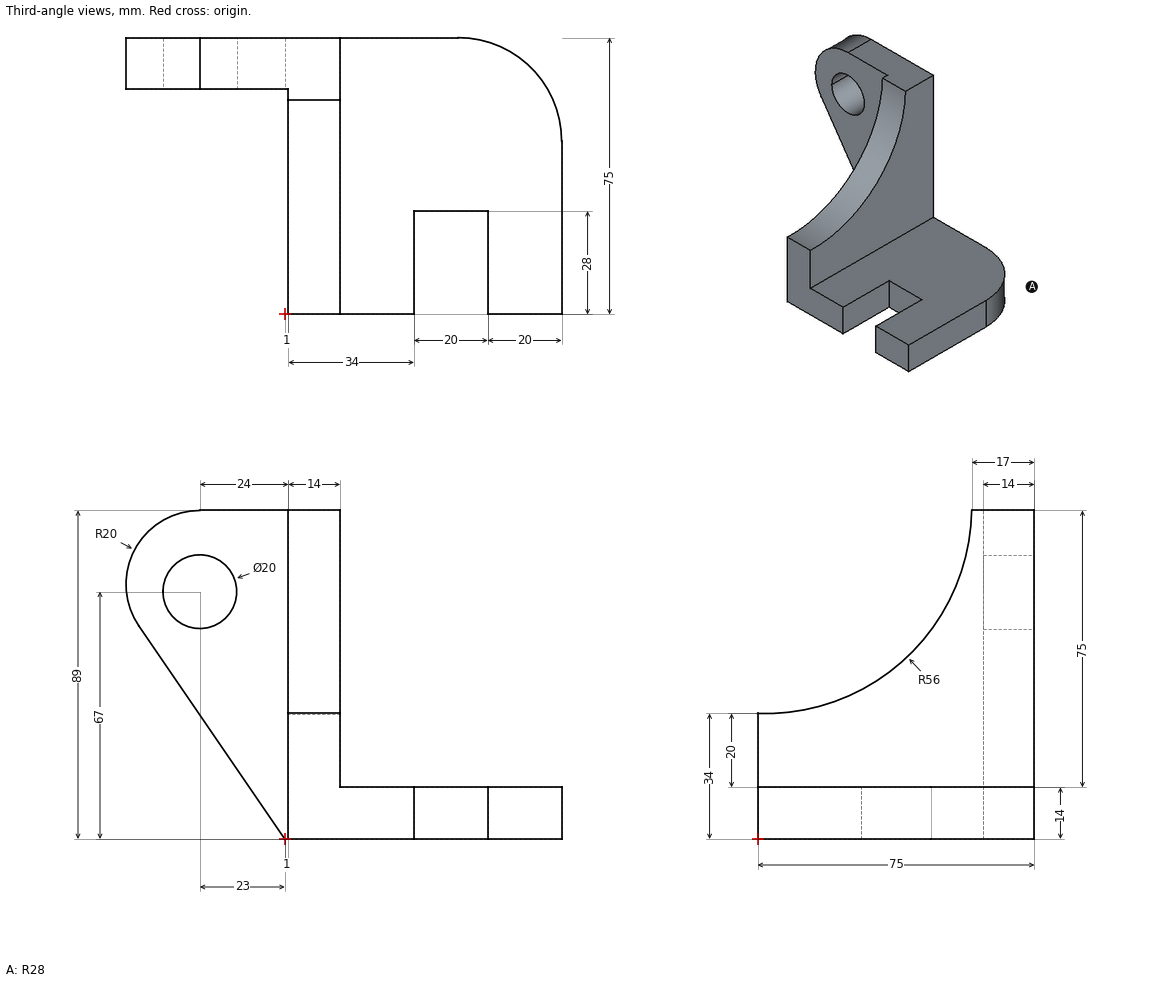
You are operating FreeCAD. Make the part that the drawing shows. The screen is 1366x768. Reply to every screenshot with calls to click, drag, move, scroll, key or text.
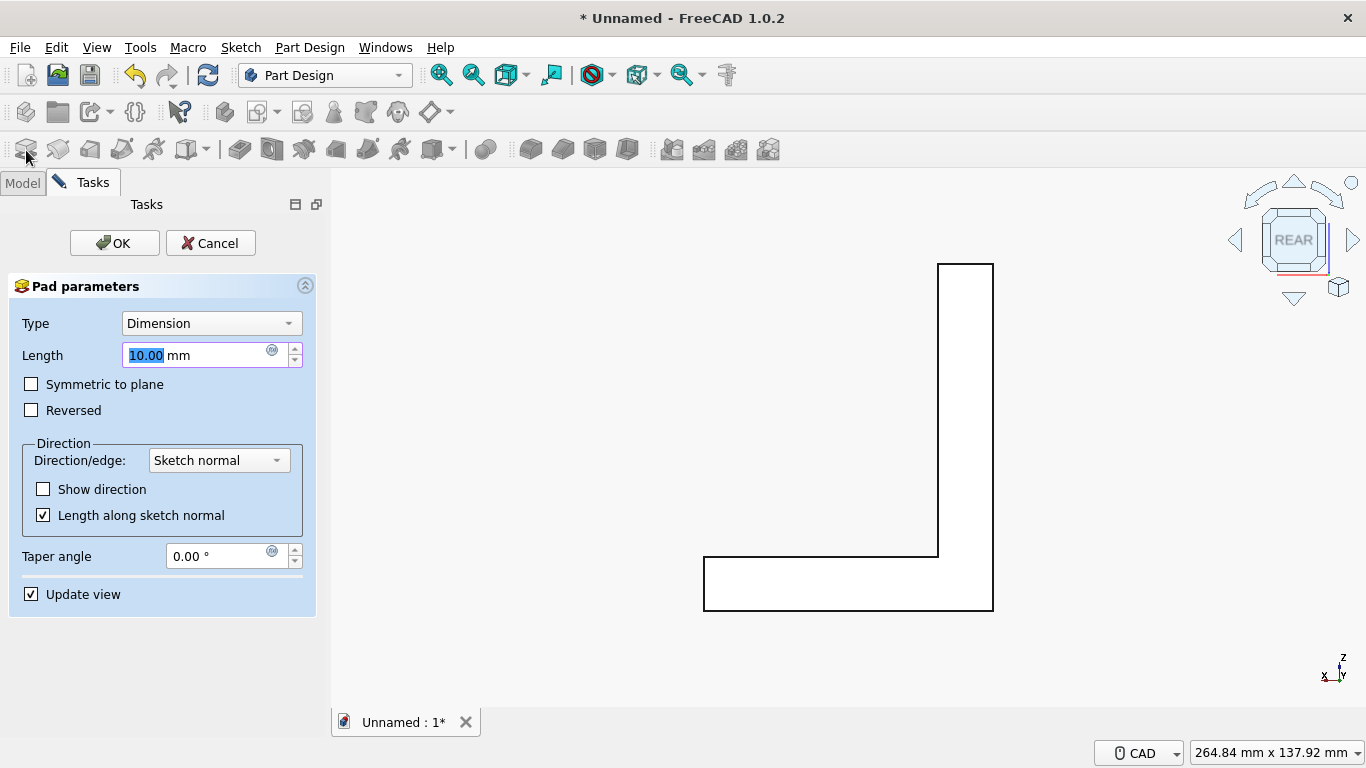
text(14)
key(Tab)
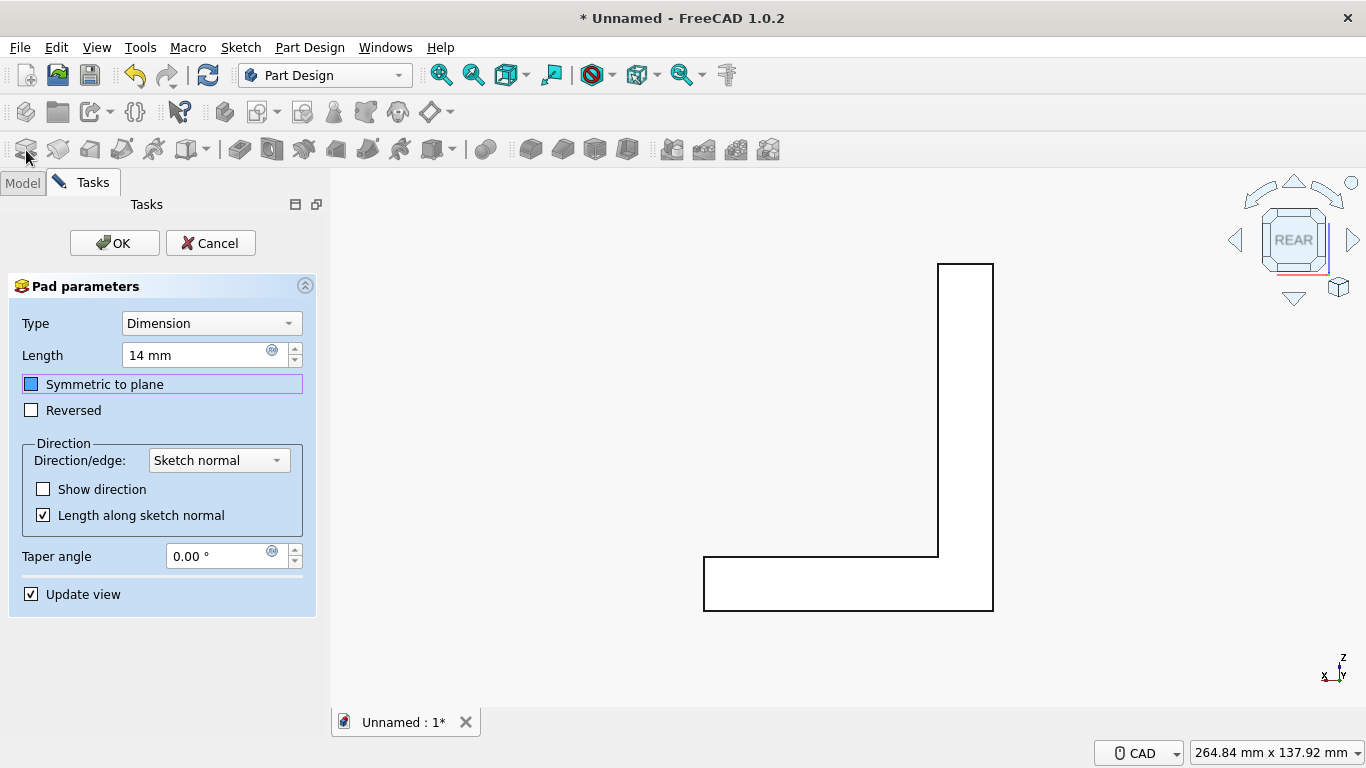
click(30, 410)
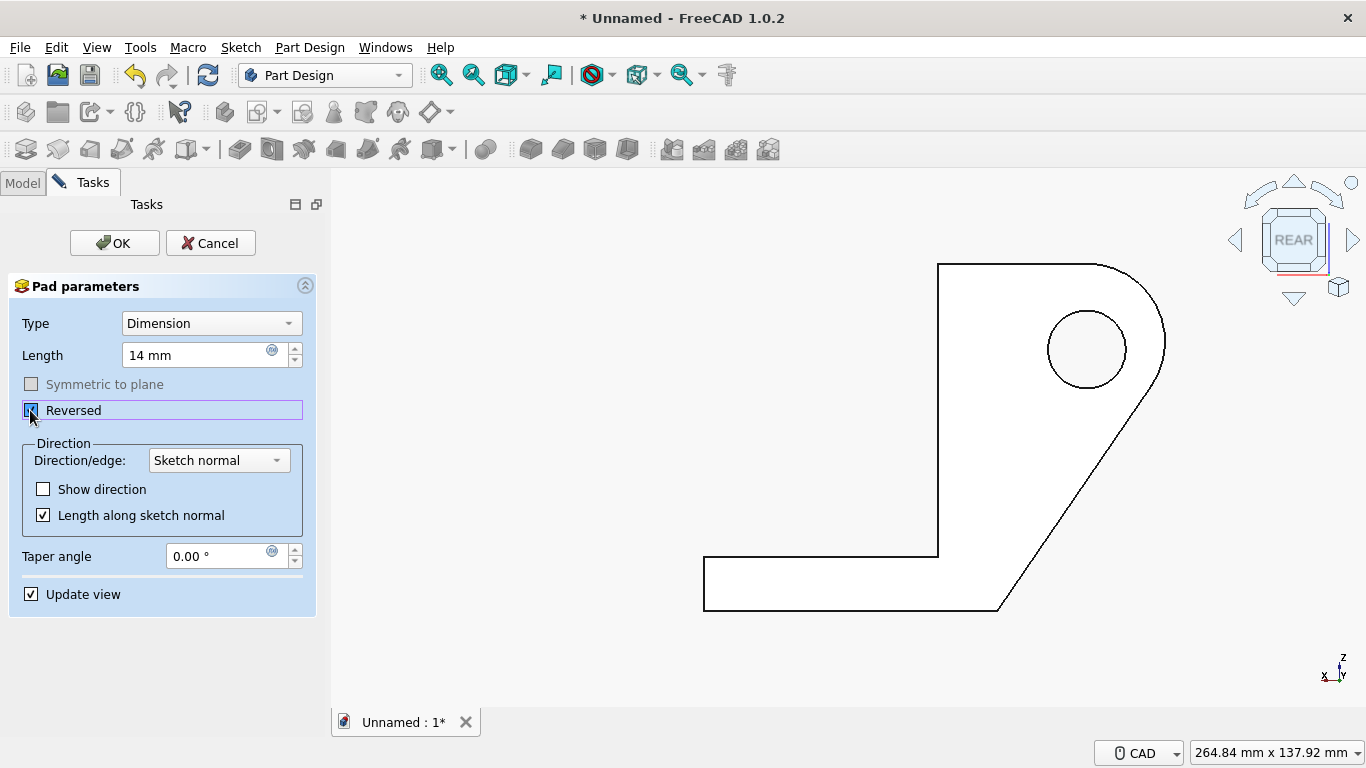
click(115, 243)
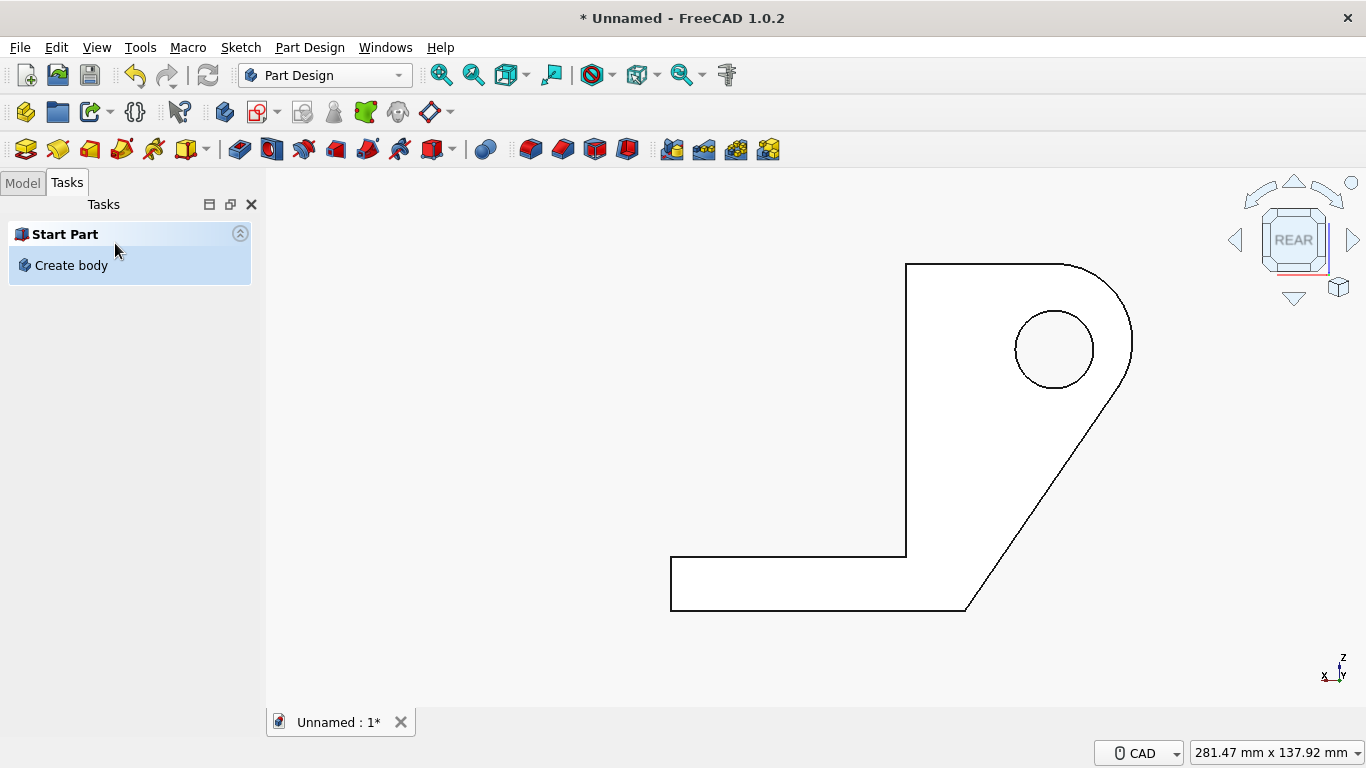
key(0)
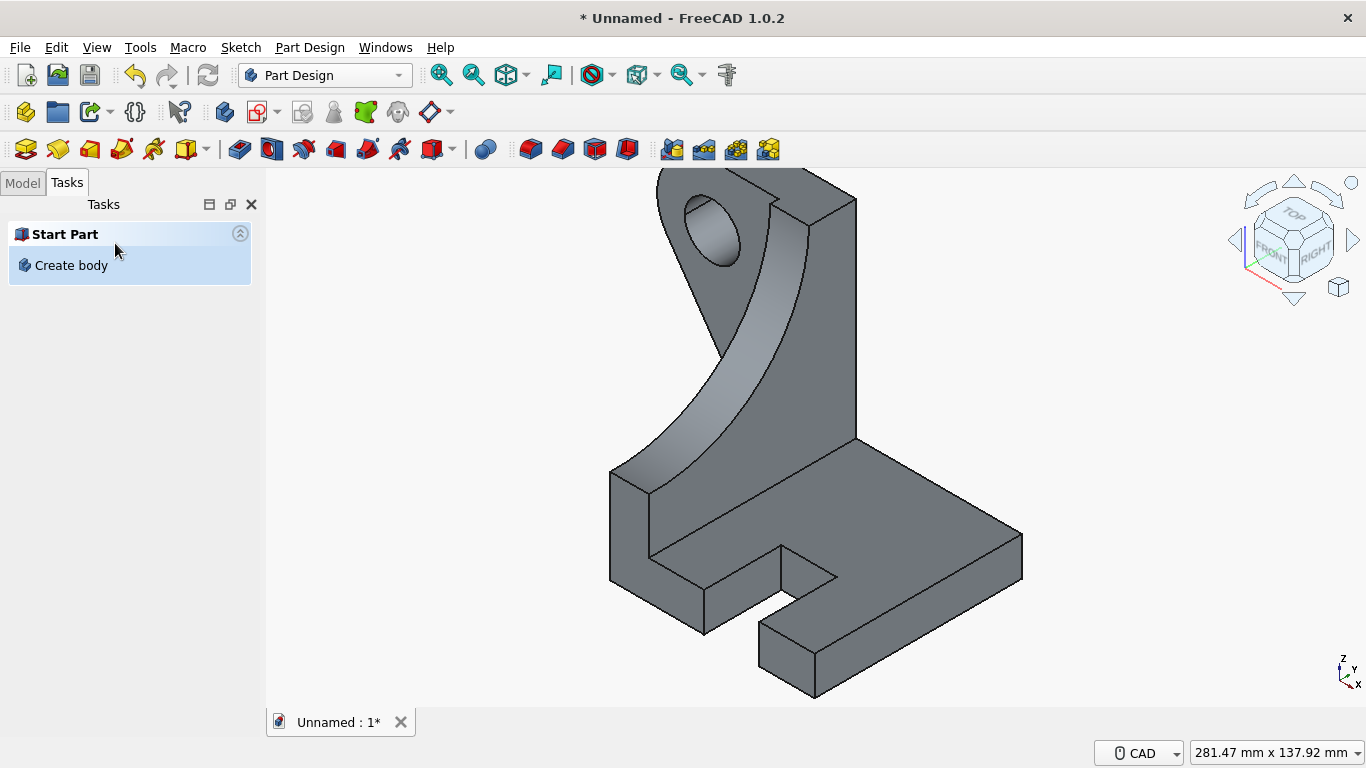
click(442, 76)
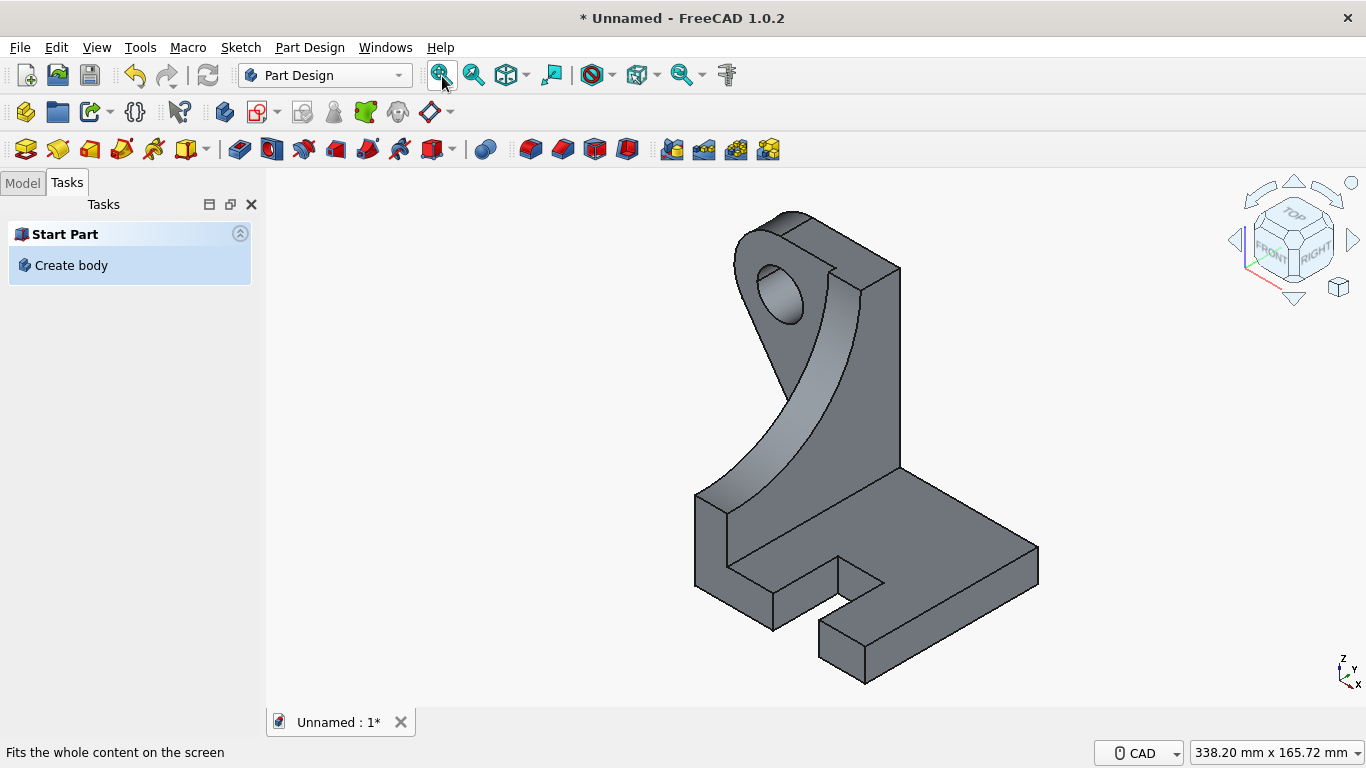
key(2)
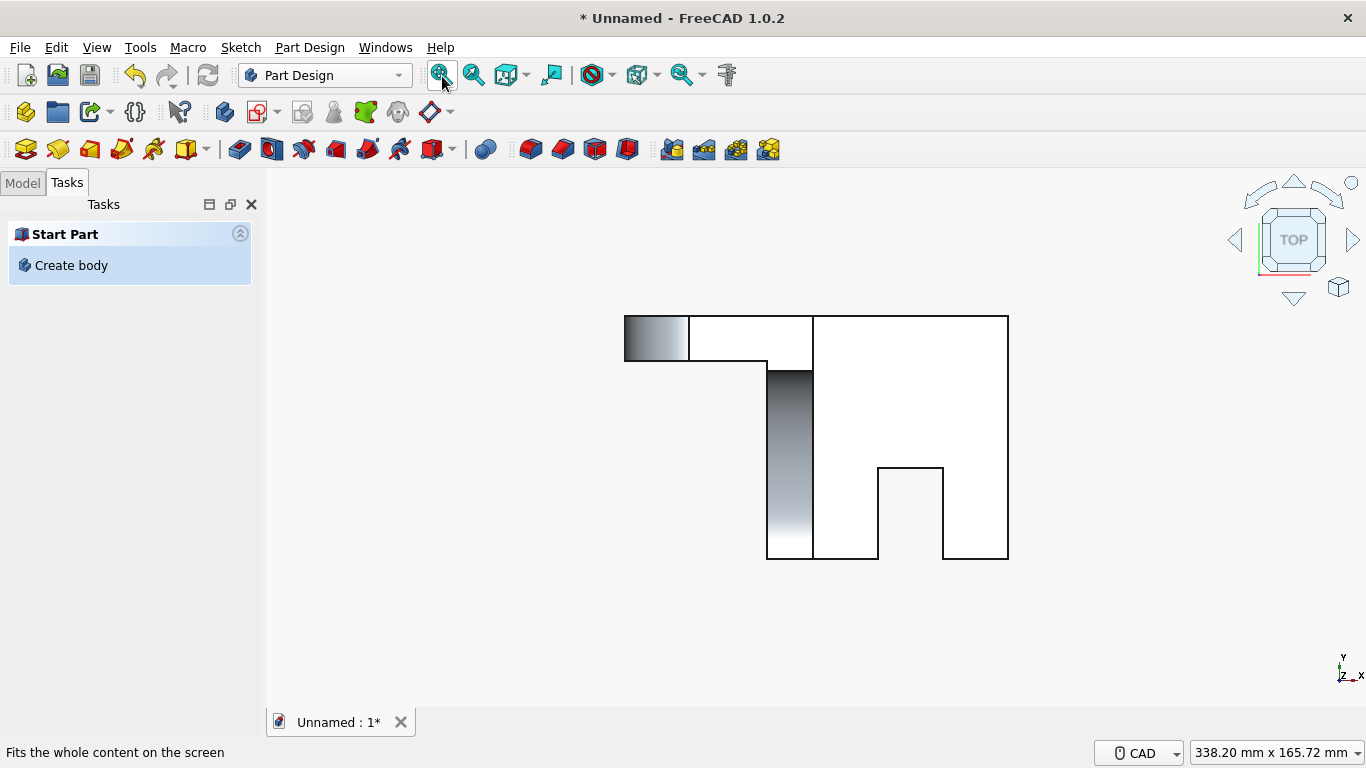
key(1)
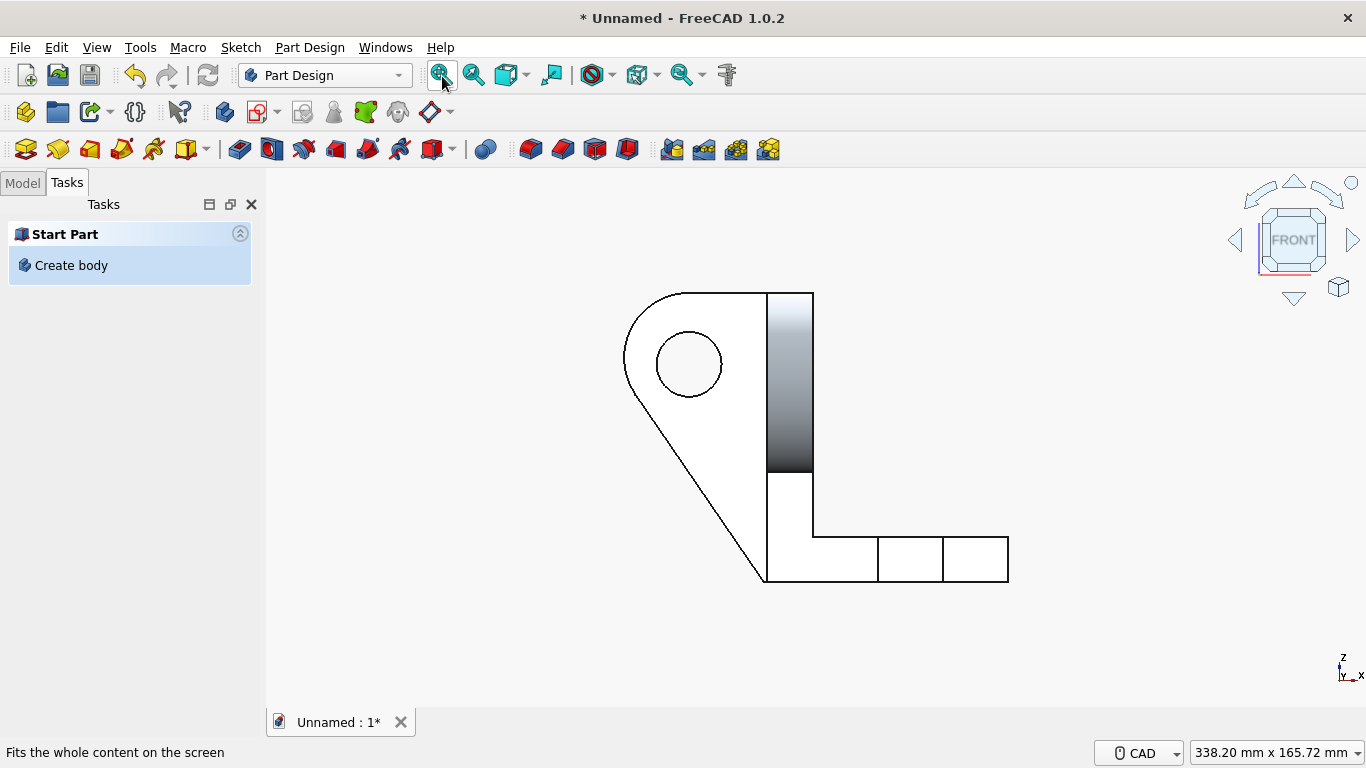
key(3)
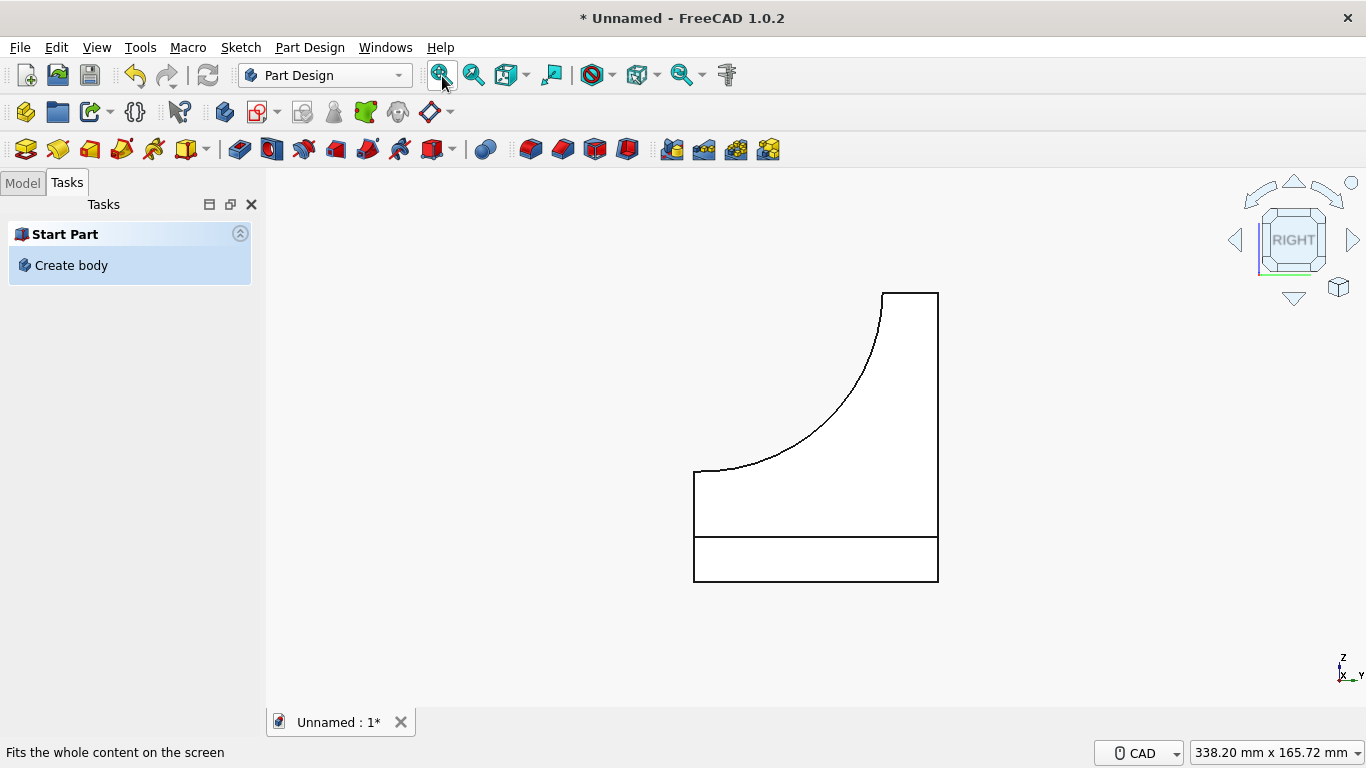
click(938, 558)